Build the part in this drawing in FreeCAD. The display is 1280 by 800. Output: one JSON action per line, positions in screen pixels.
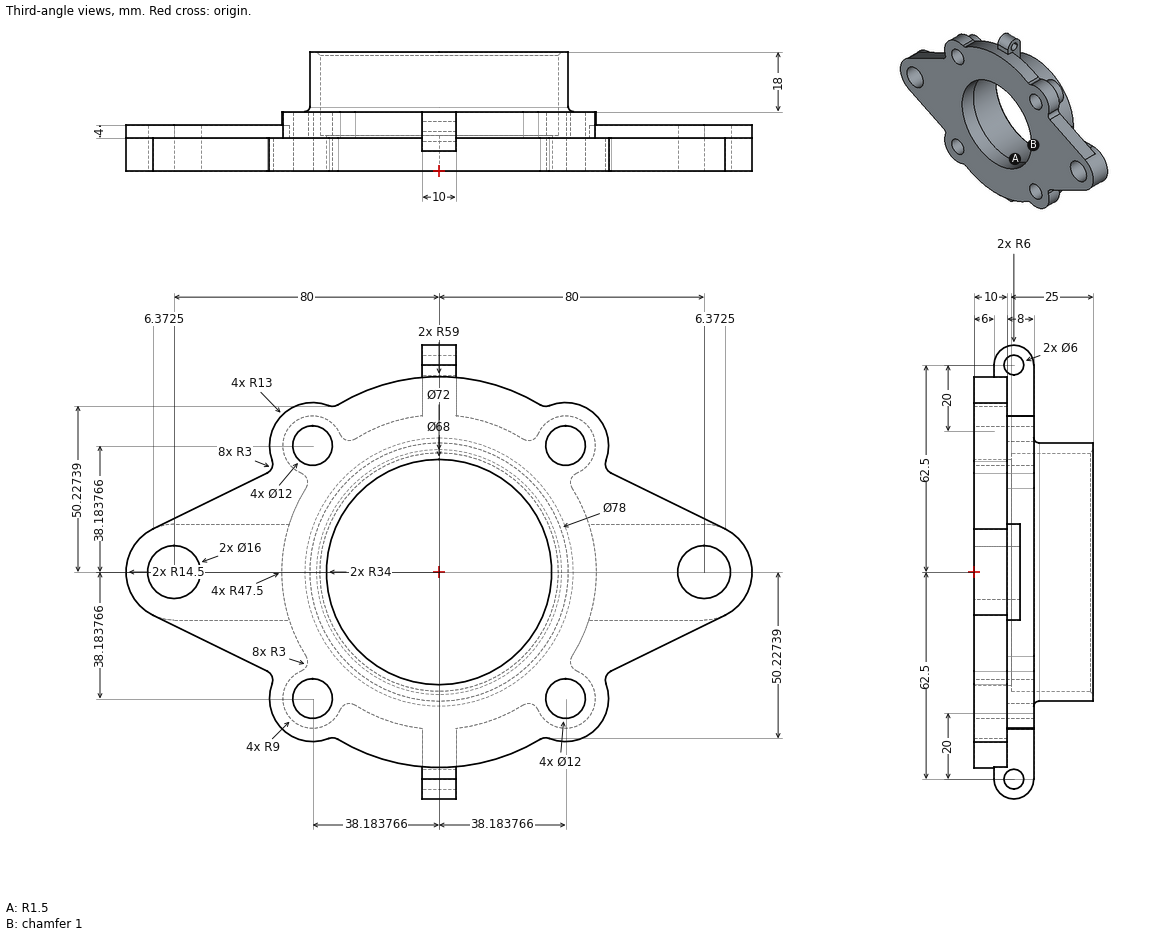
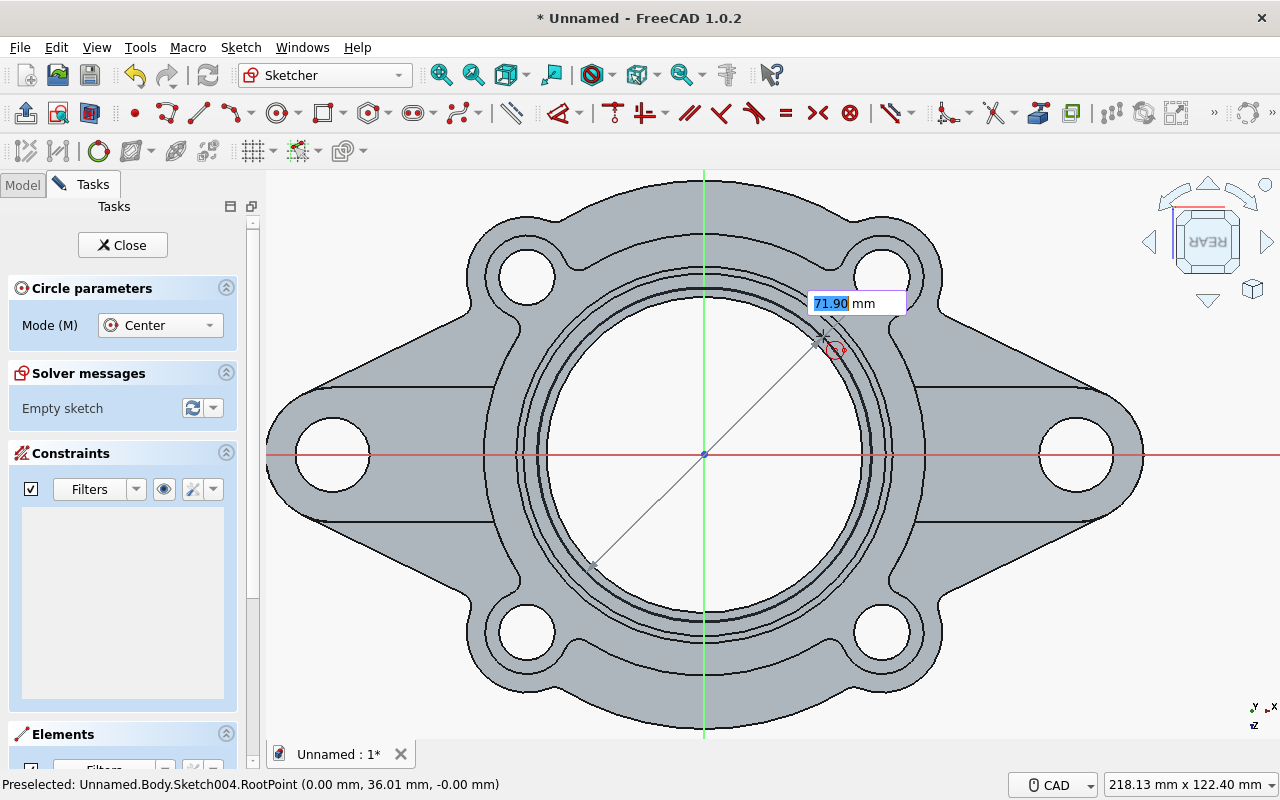
{"action": "type", "text": "72"}
{"action": "key", "text": "Return"}
{"action": "key", "text": "Escape"}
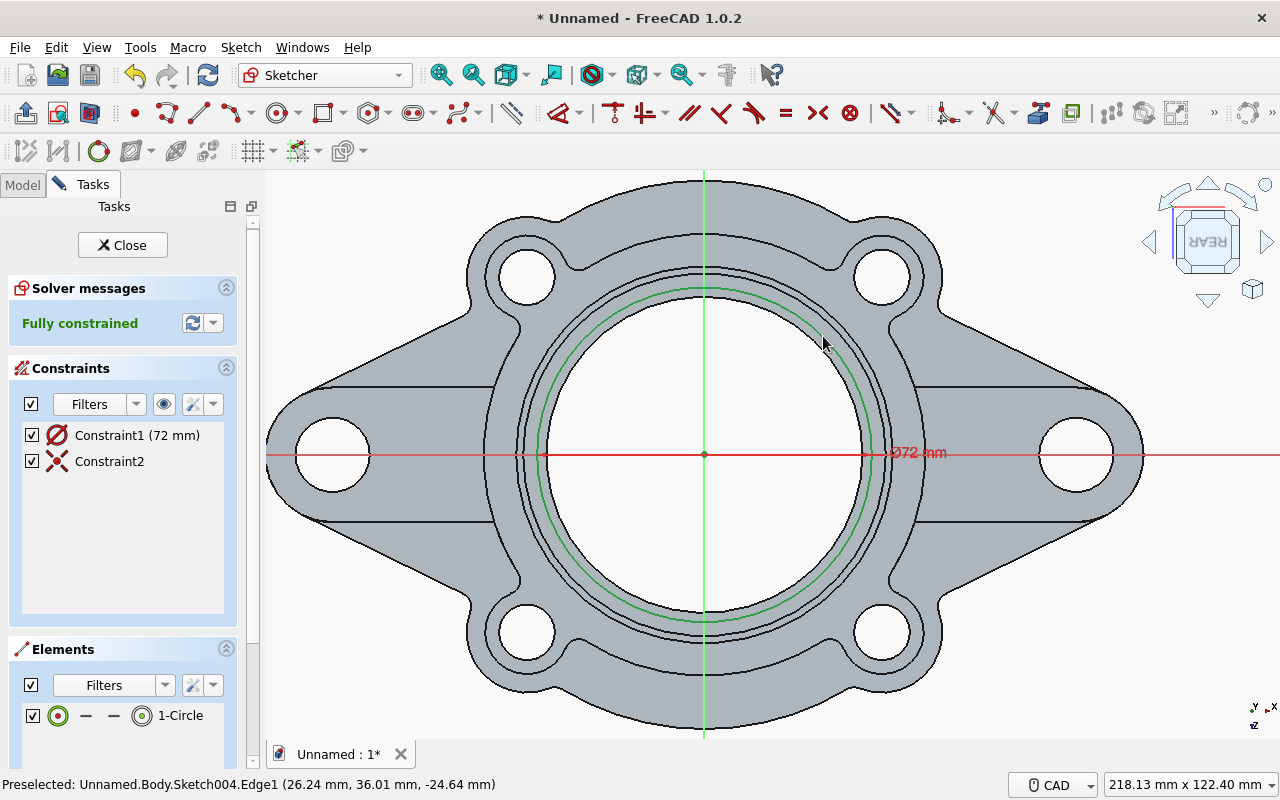
{"action": "left_click", "coordinate": [123, 245]}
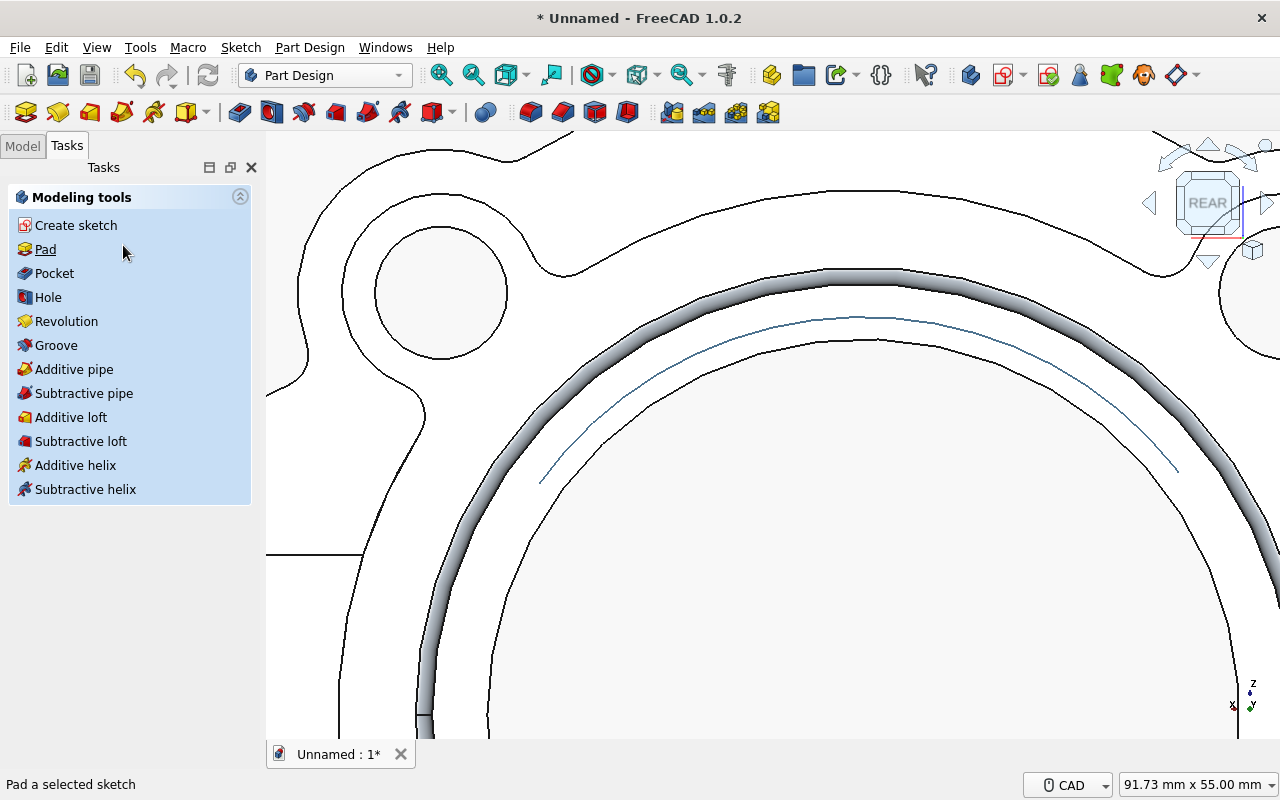
{"action": "left_click", "coordinate": [240, 112]}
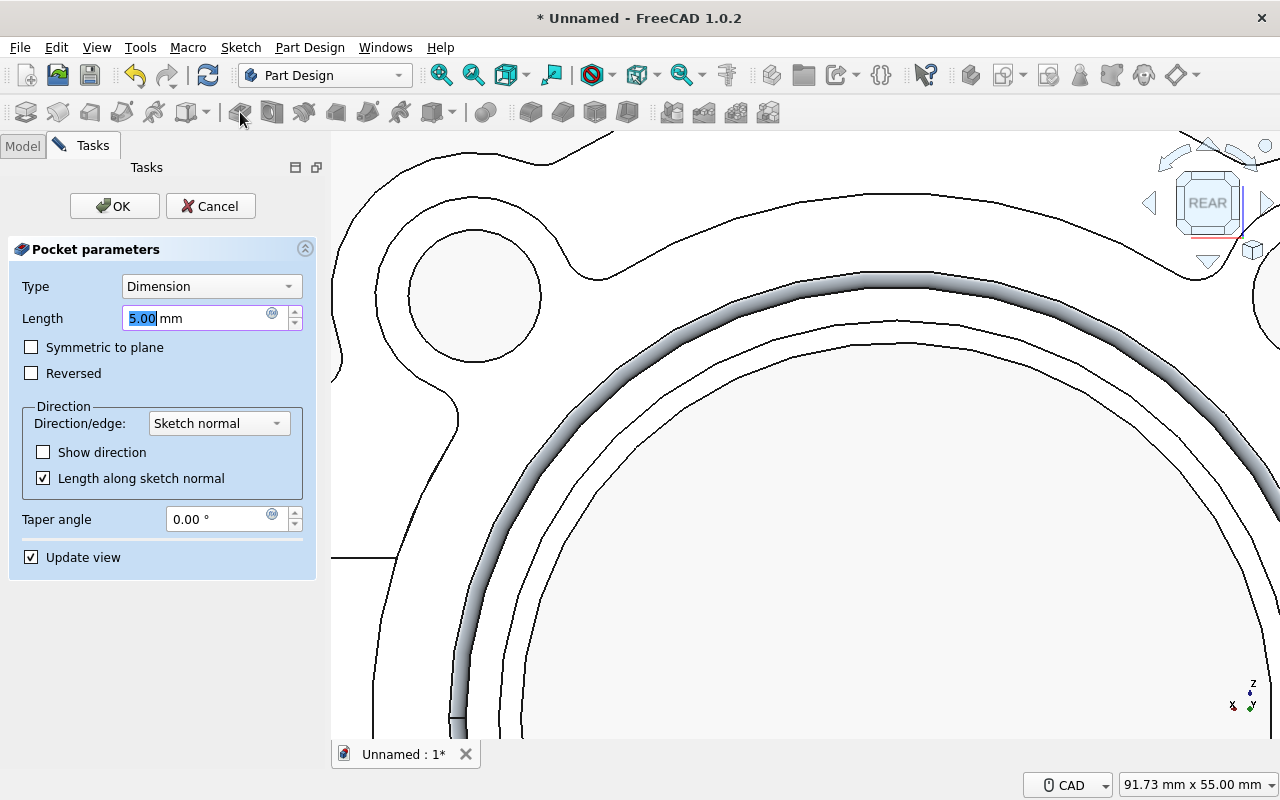
{"action": "type", "text": "25"}
{"action": "key", "text": "Tab"}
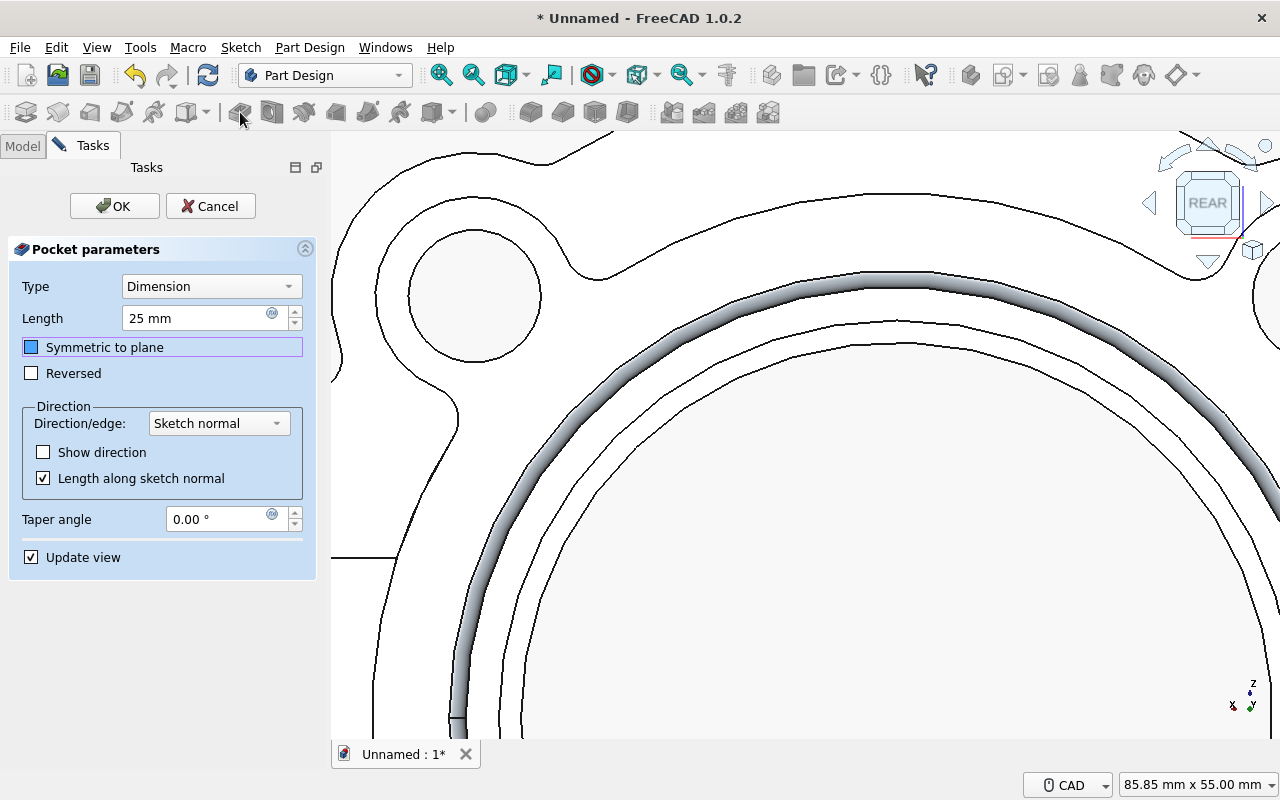
{"action": "left_click", "coordinate": [115, 206]}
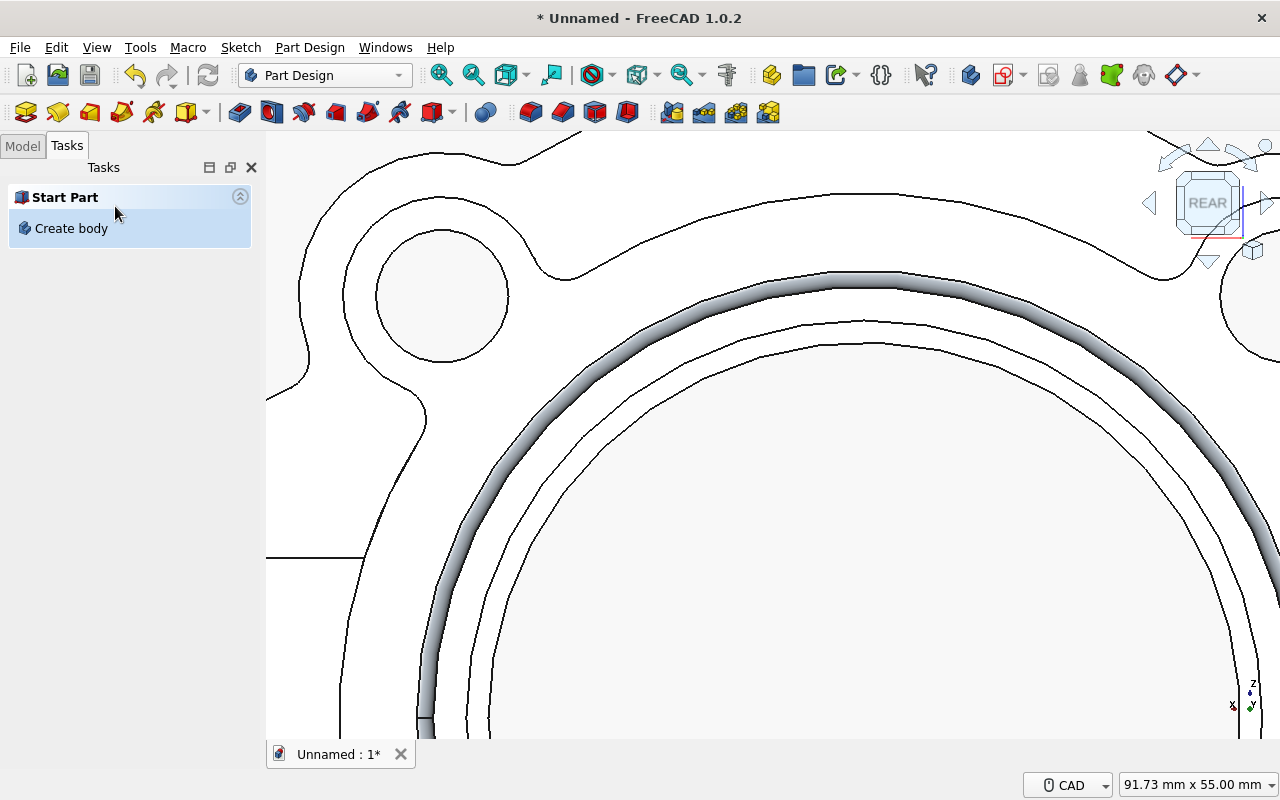
{"action": "left_click", "coordinate": [442, 76]}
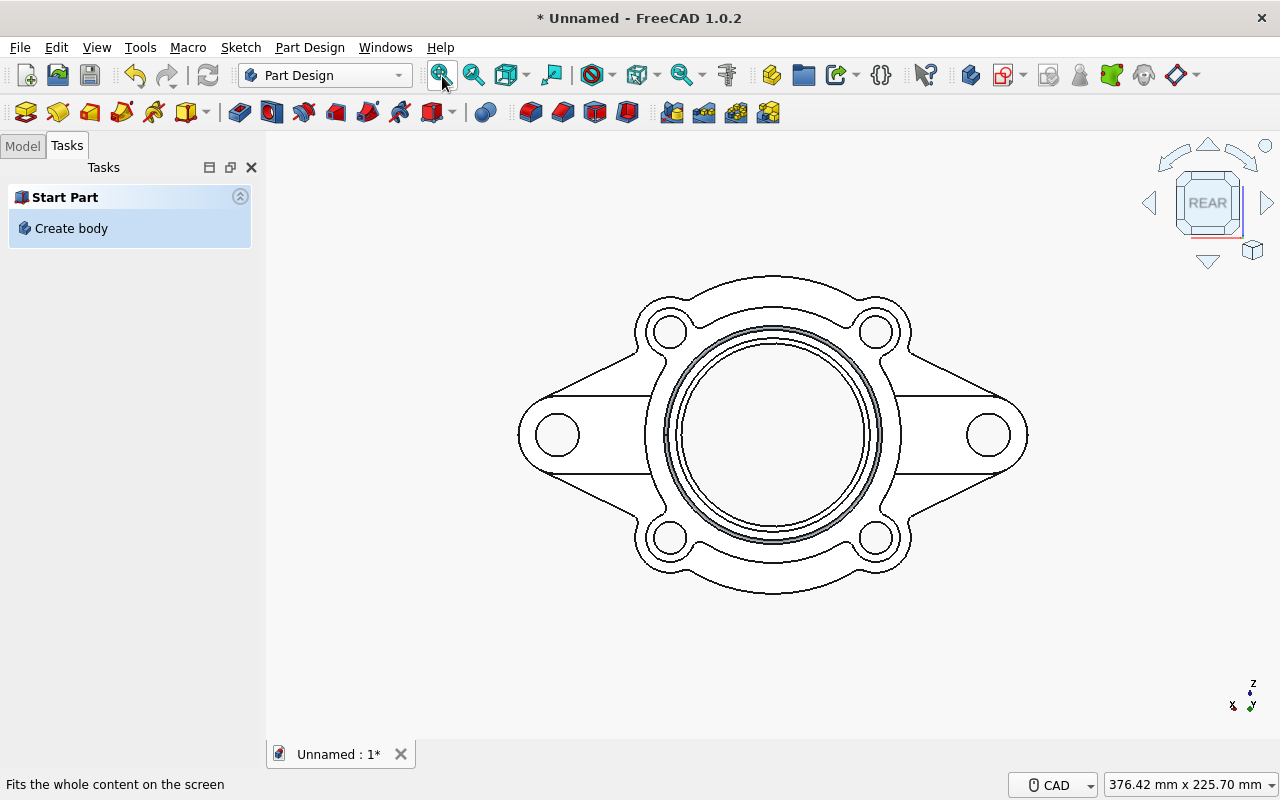
{"action": "left_click", "coordinate": [851, 377]}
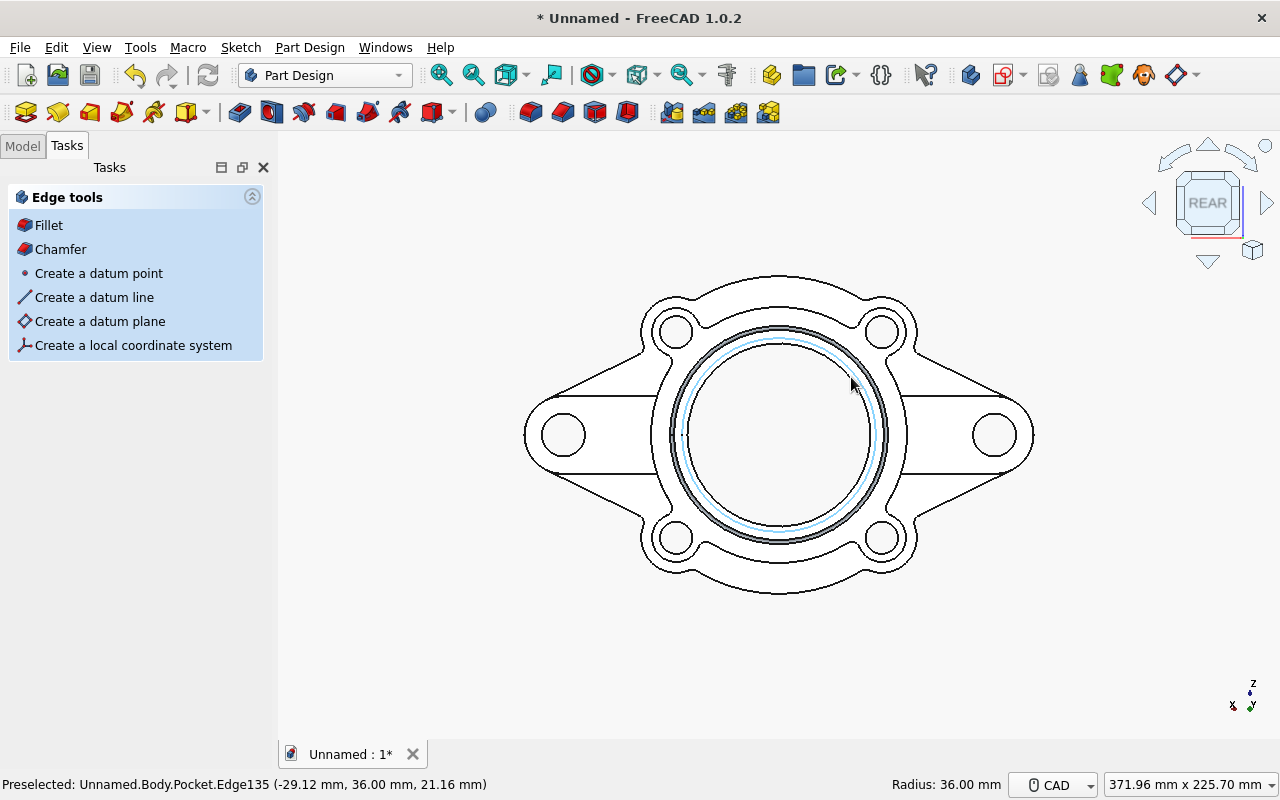
{"action": "left_click", "coordinate": [564, 112]}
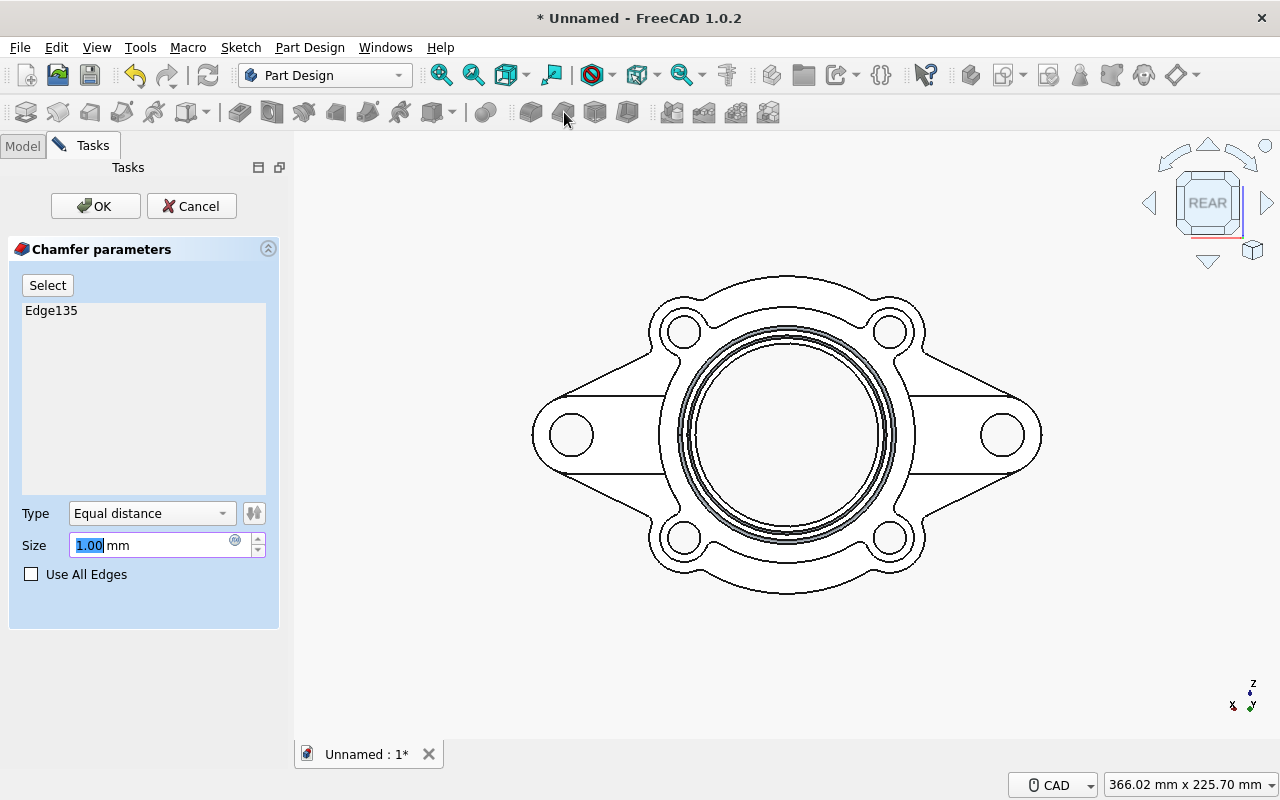
{"action": "type", "text": "1"}
{"action": "key", "text": "Tab"}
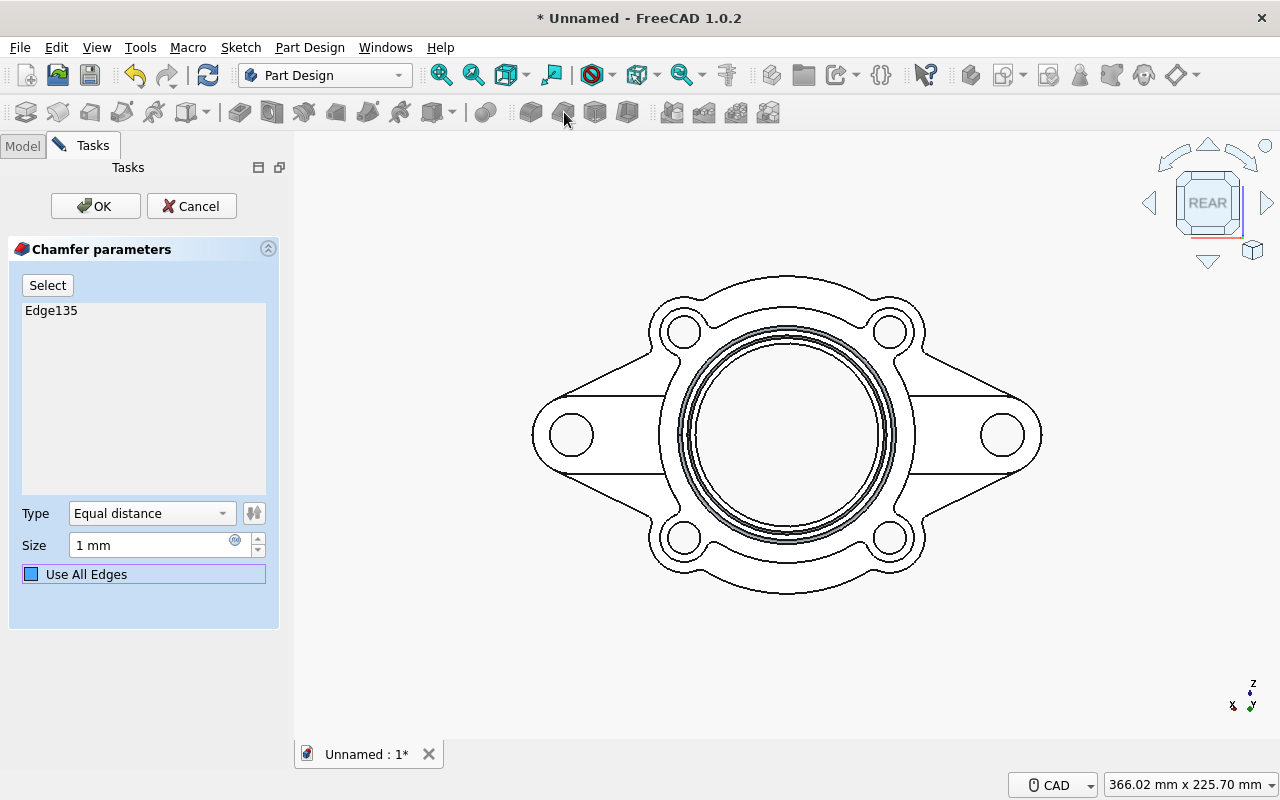
{"action": "left_click", "coordinate": [96, 206]}